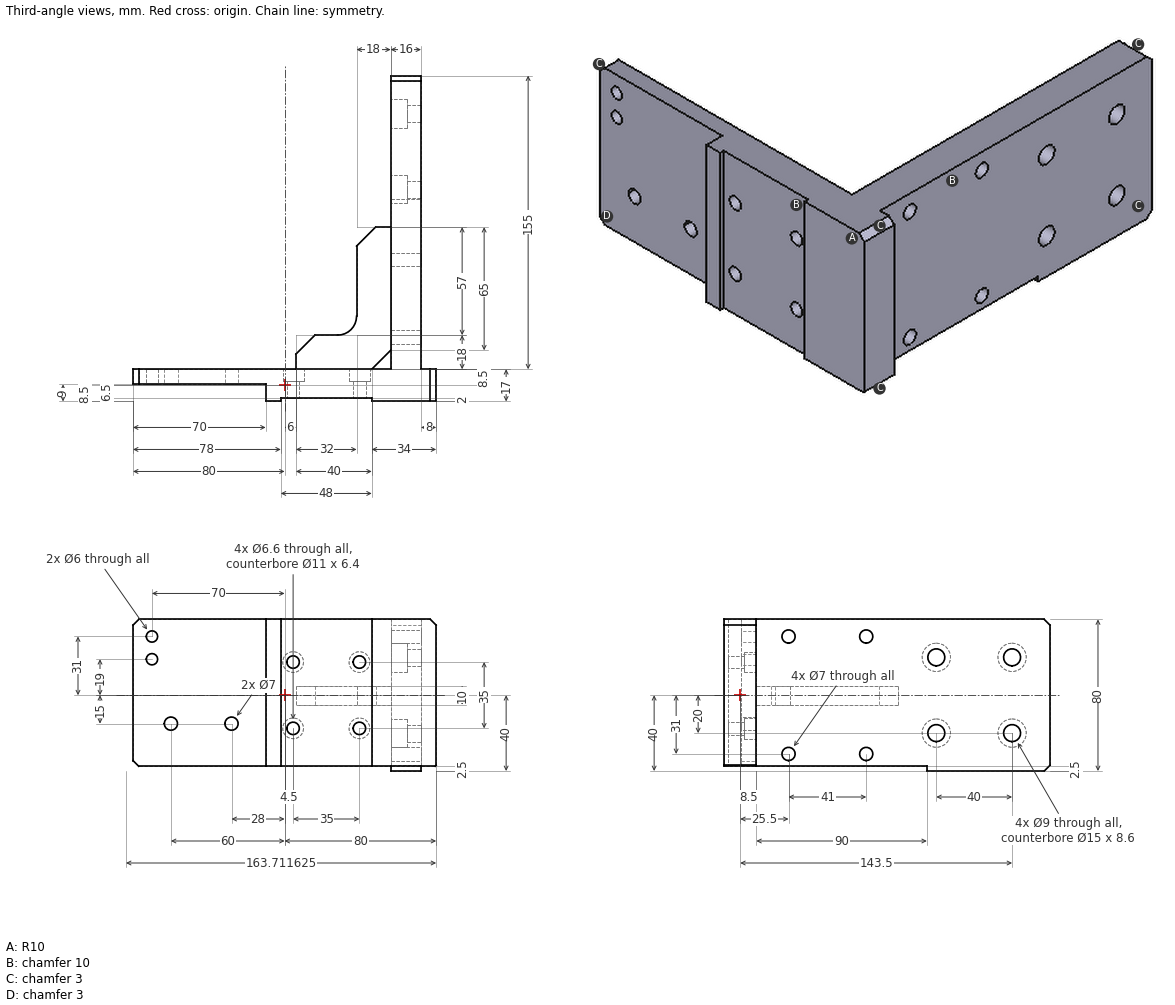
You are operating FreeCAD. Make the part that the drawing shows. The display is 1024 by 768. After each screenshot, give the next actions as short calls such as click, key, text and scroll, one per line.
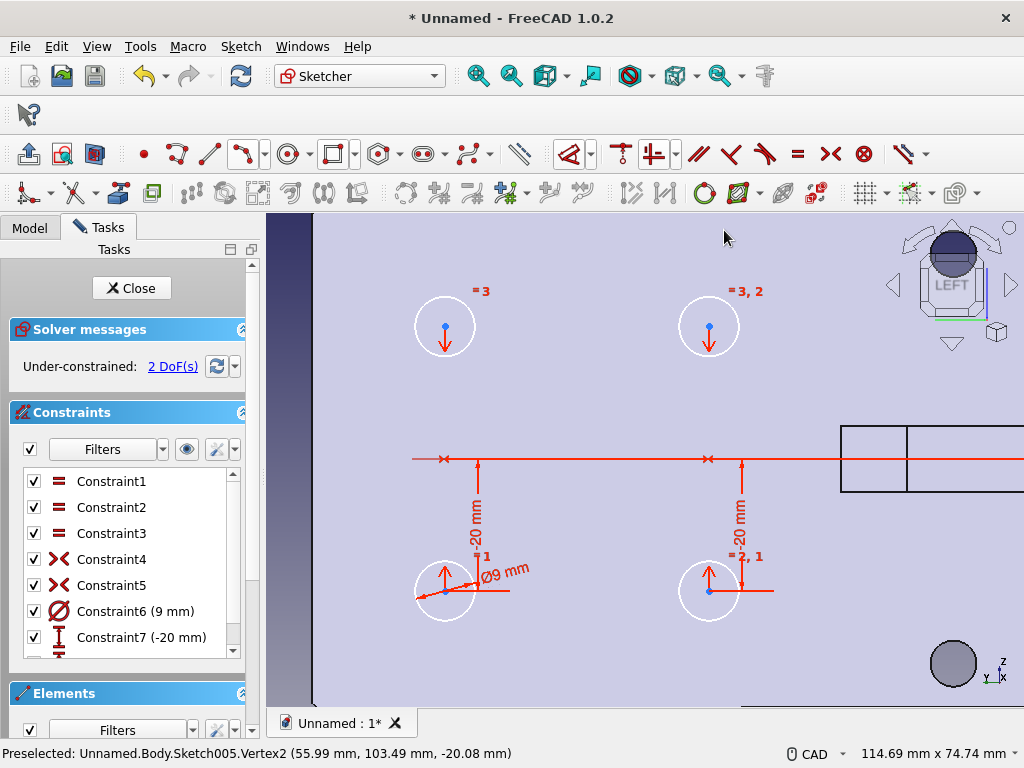
click(445, 591)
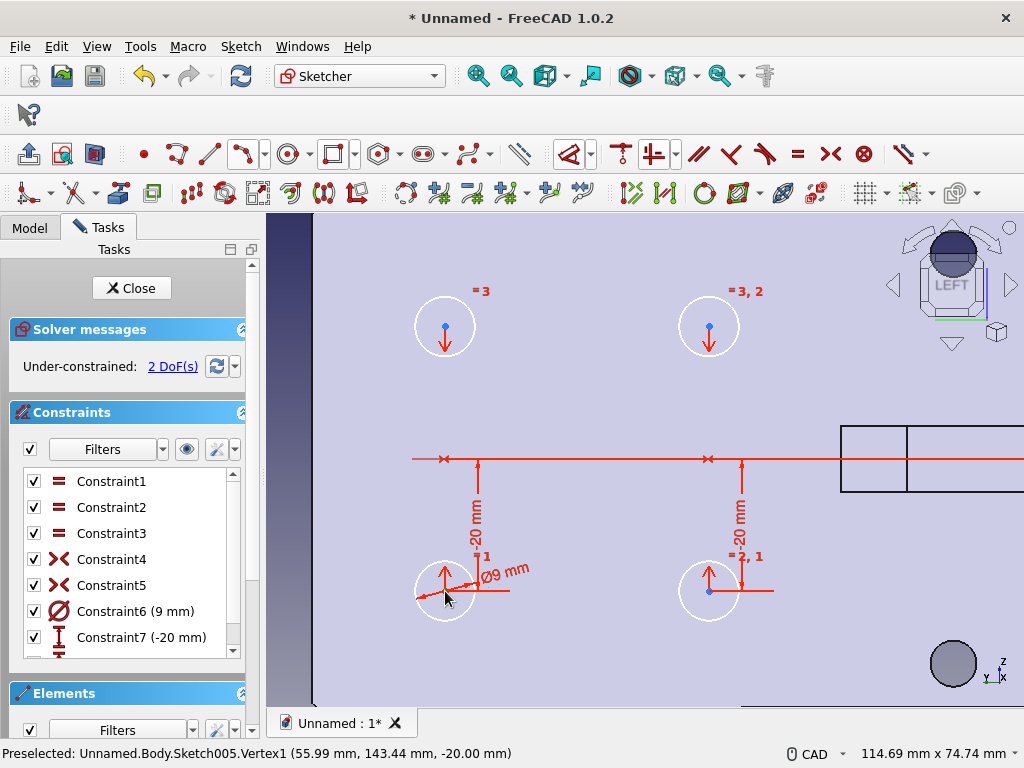
click(709, 591)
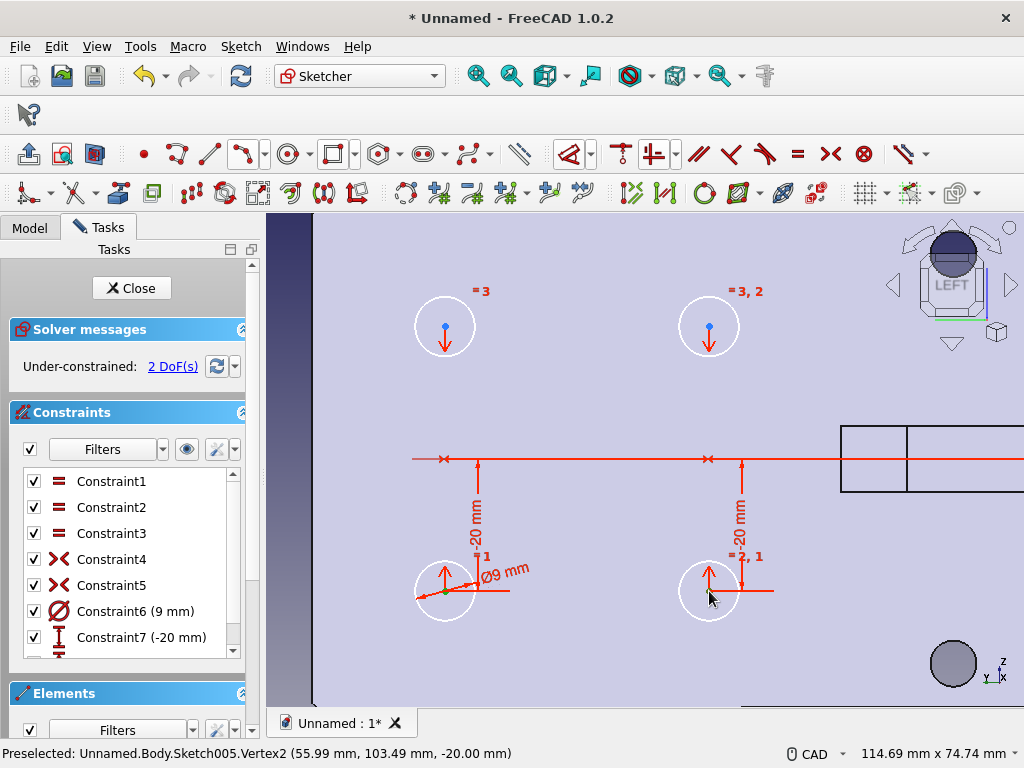
key(l)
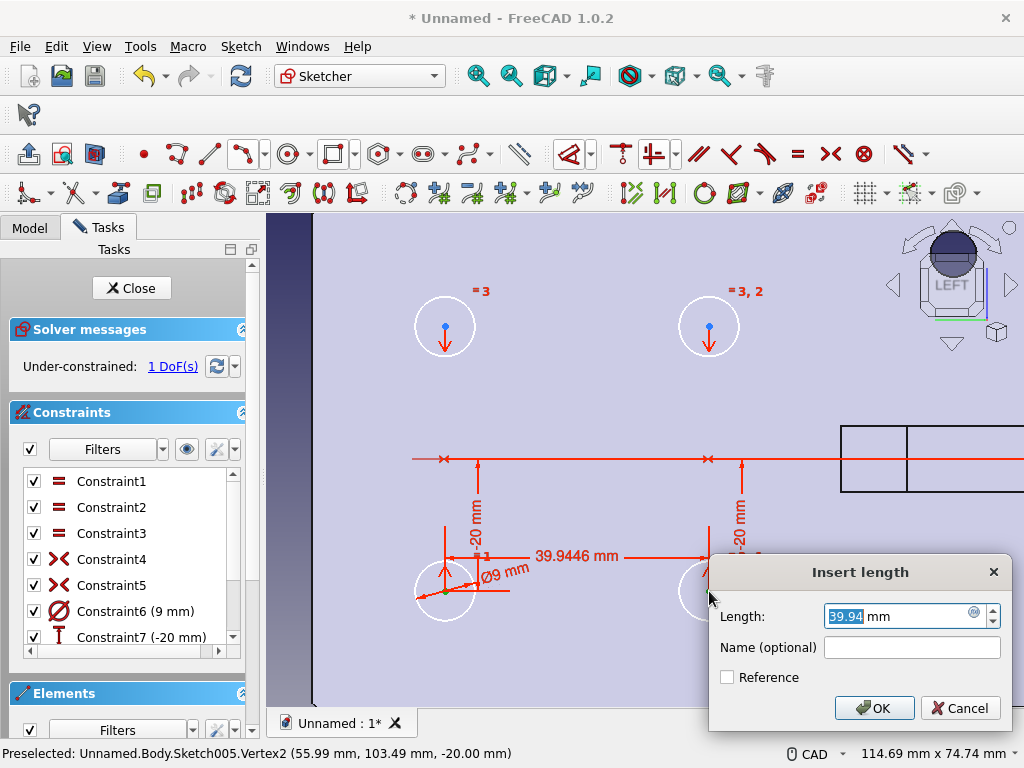
text(40)
key(Return)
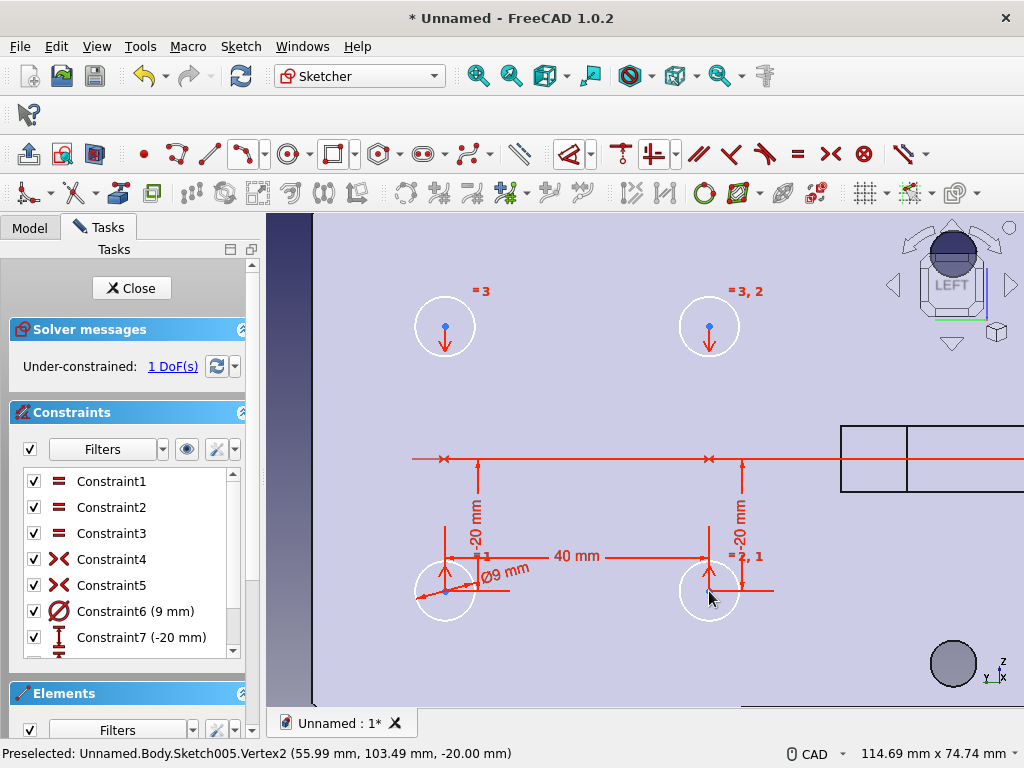
click(445, 591)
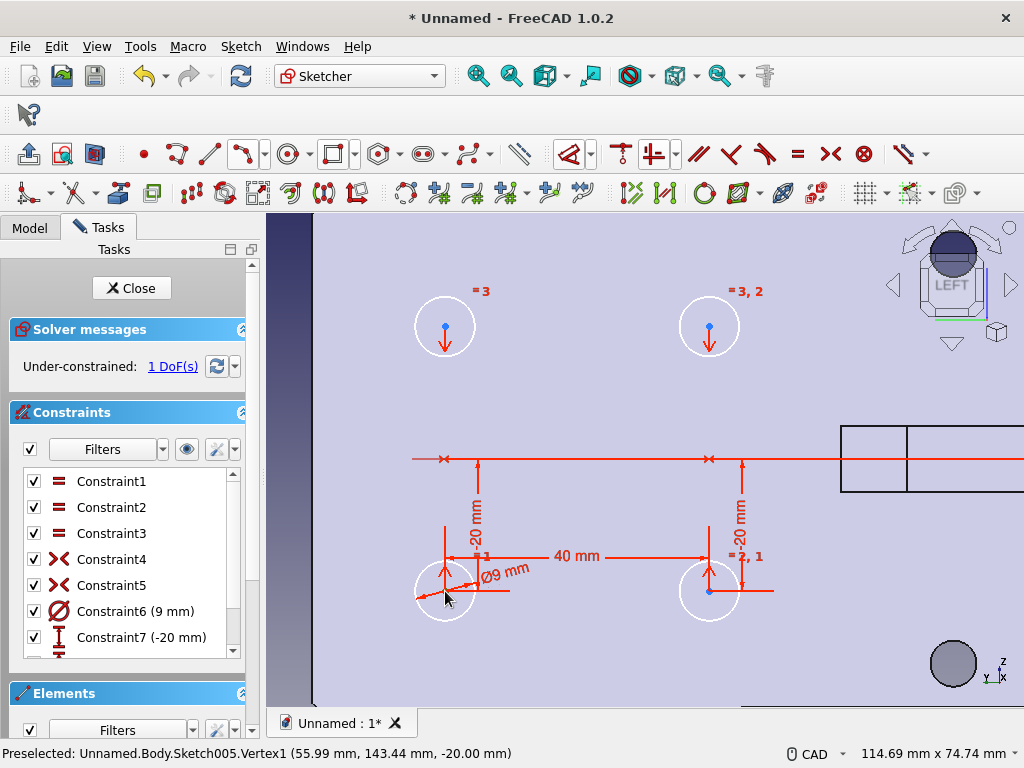
click(590, 154)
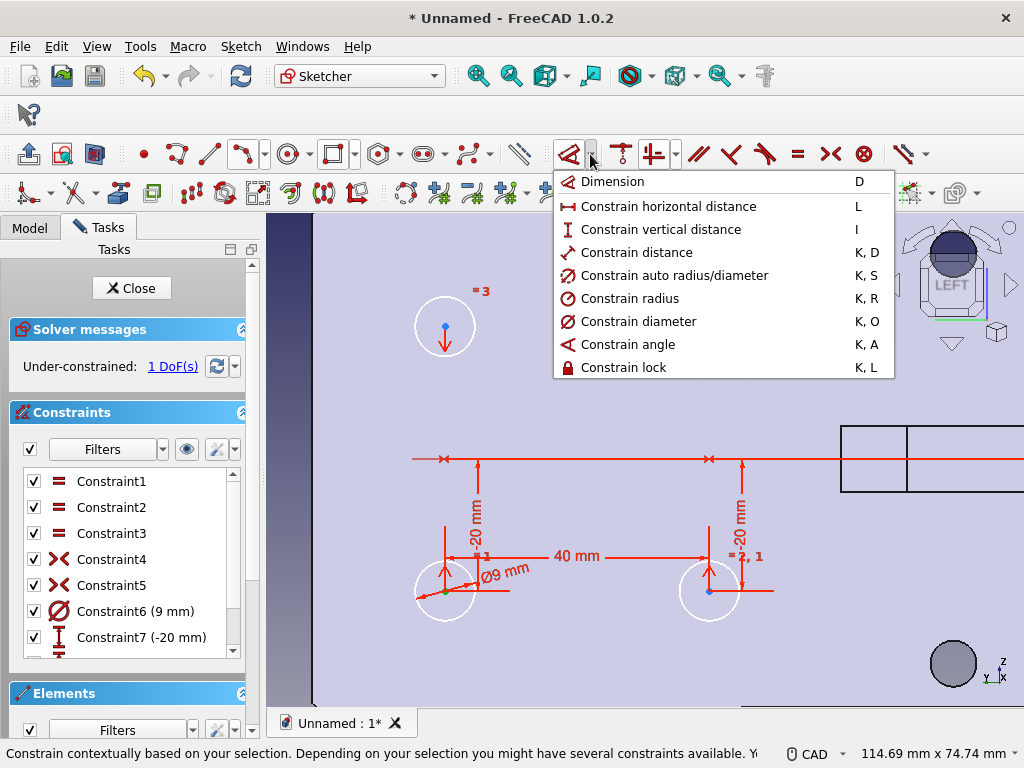
click(724, 206)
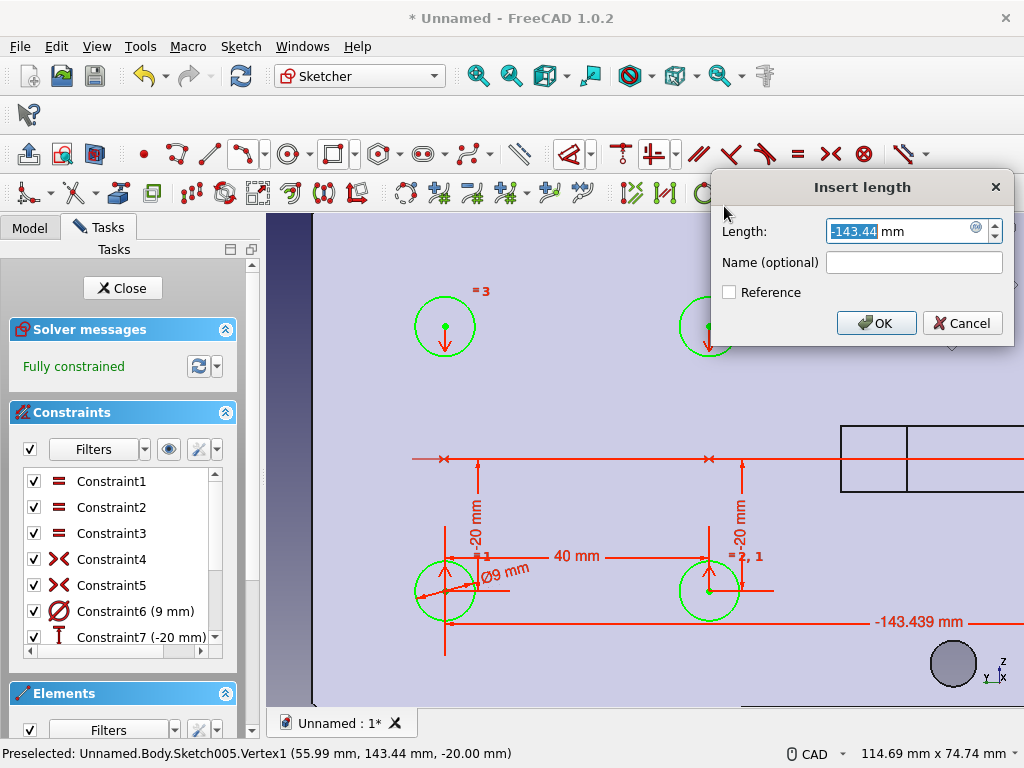
text(-143.5)
key(Return)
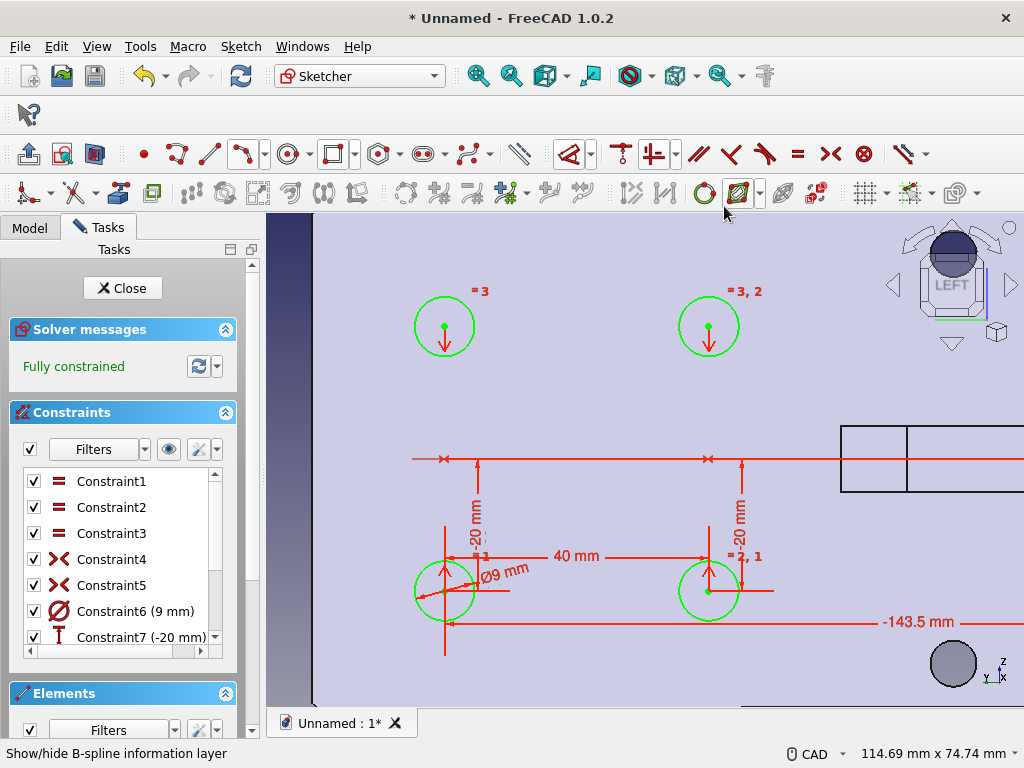
click(123, 288)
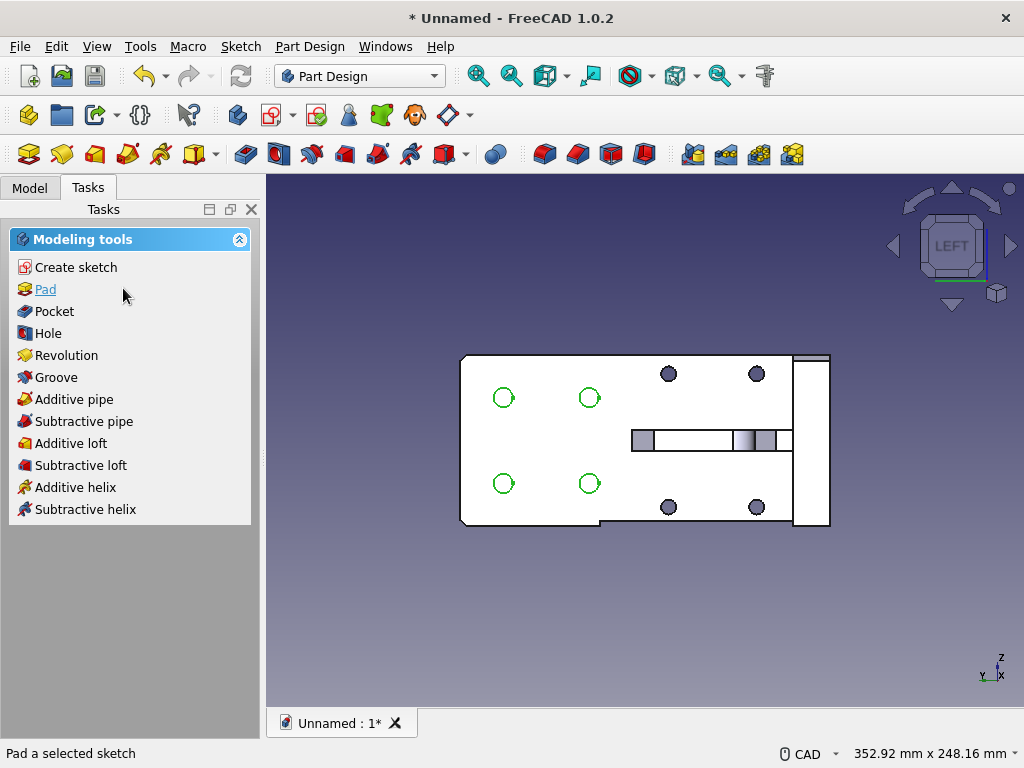
click(279, 154)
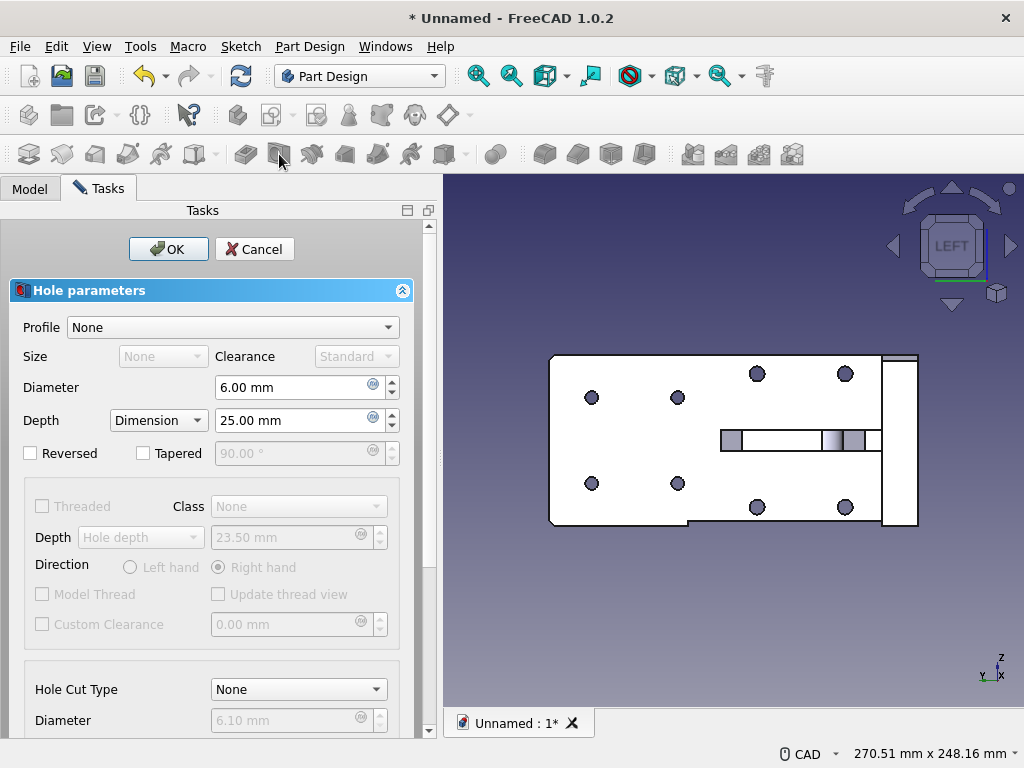
triple_click(300, 388)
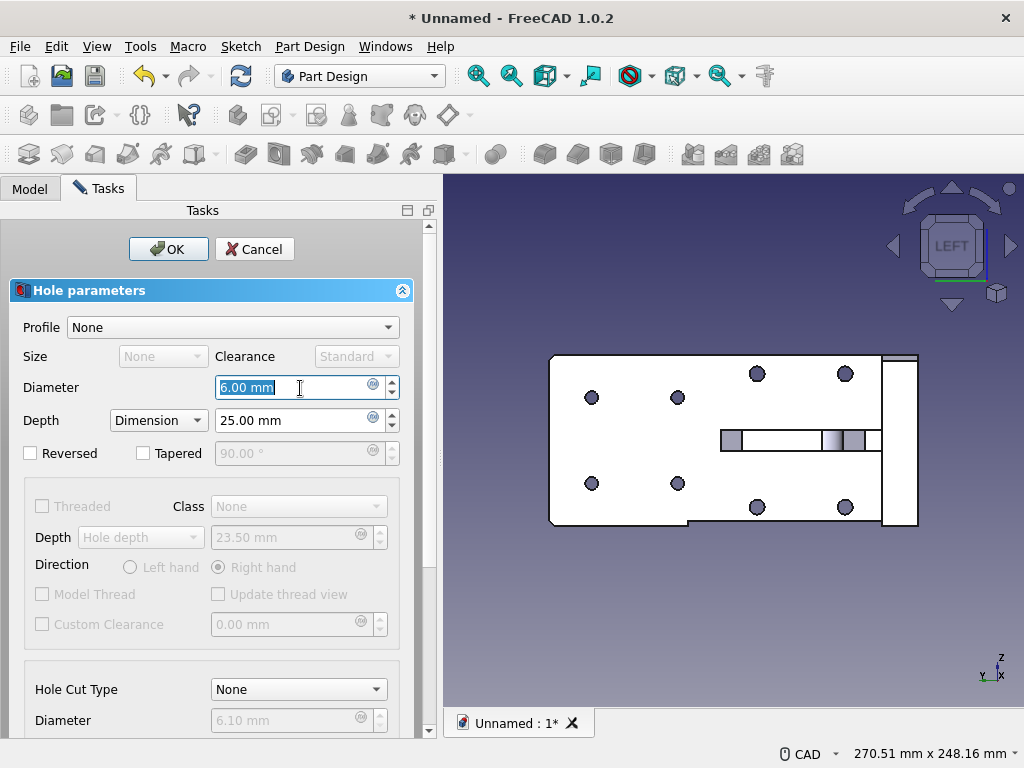
text(9)
key(Tab)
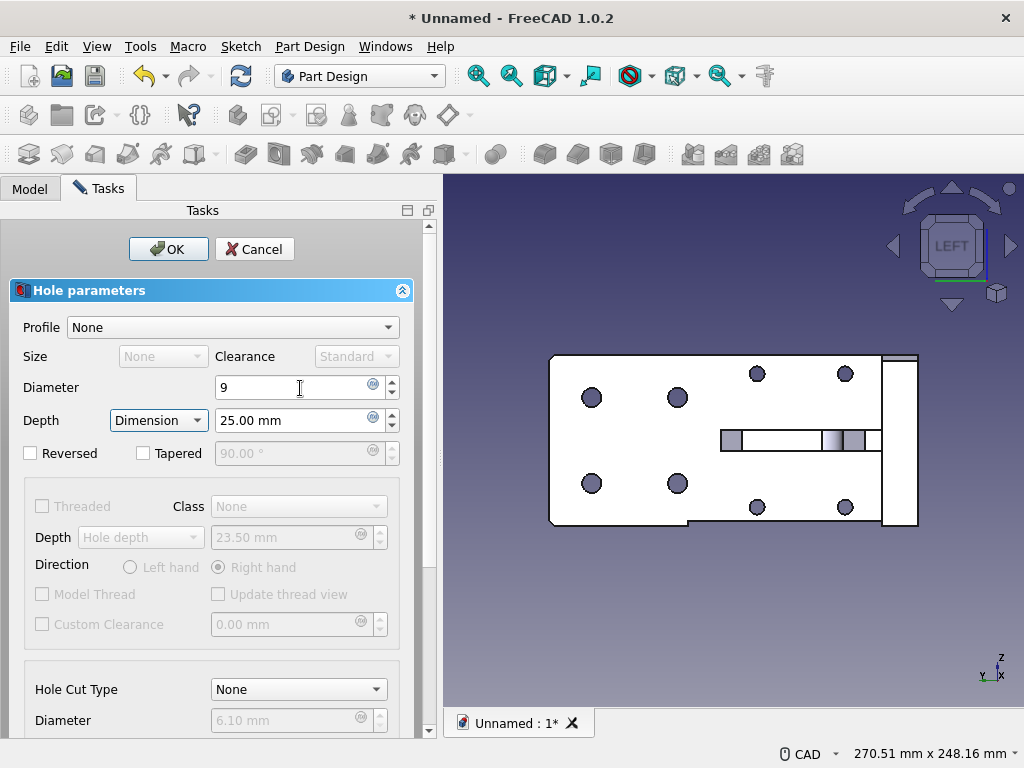
click(160, 420)